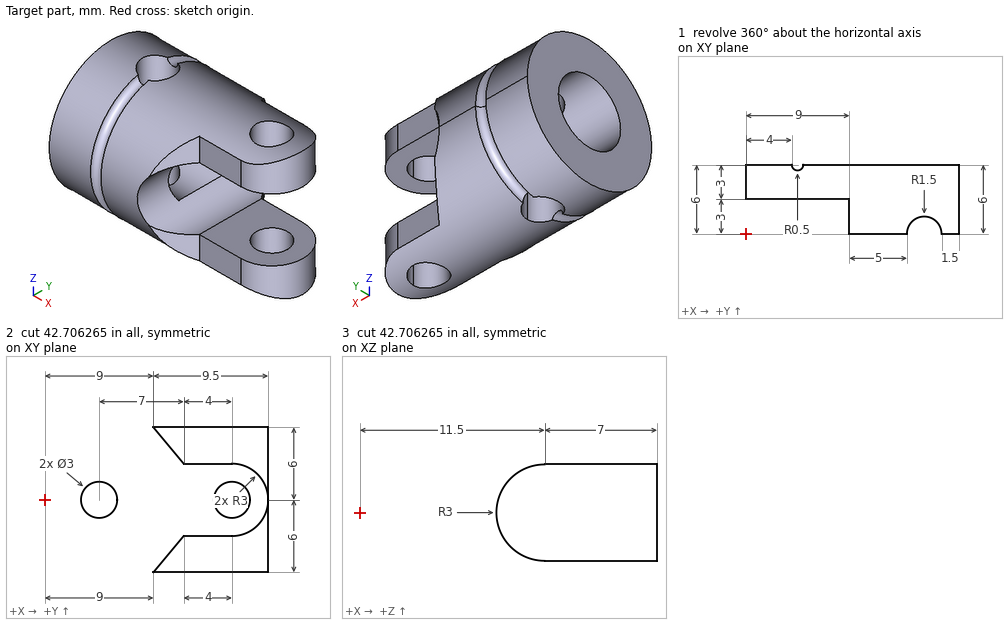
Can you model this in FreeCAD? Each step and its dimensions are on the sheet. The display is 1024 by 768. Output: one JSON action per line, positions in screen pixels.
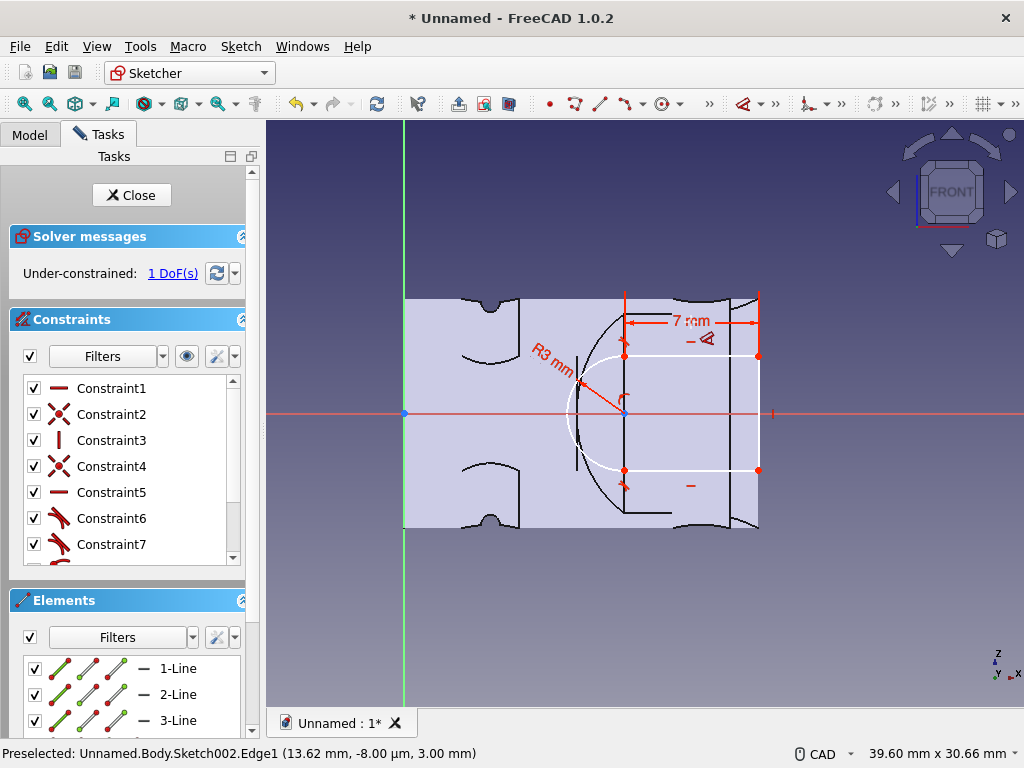
{"action": "left_click", "coordinate": [625, 356]}
{"action": "left_click", "coordinate": [515, 322]}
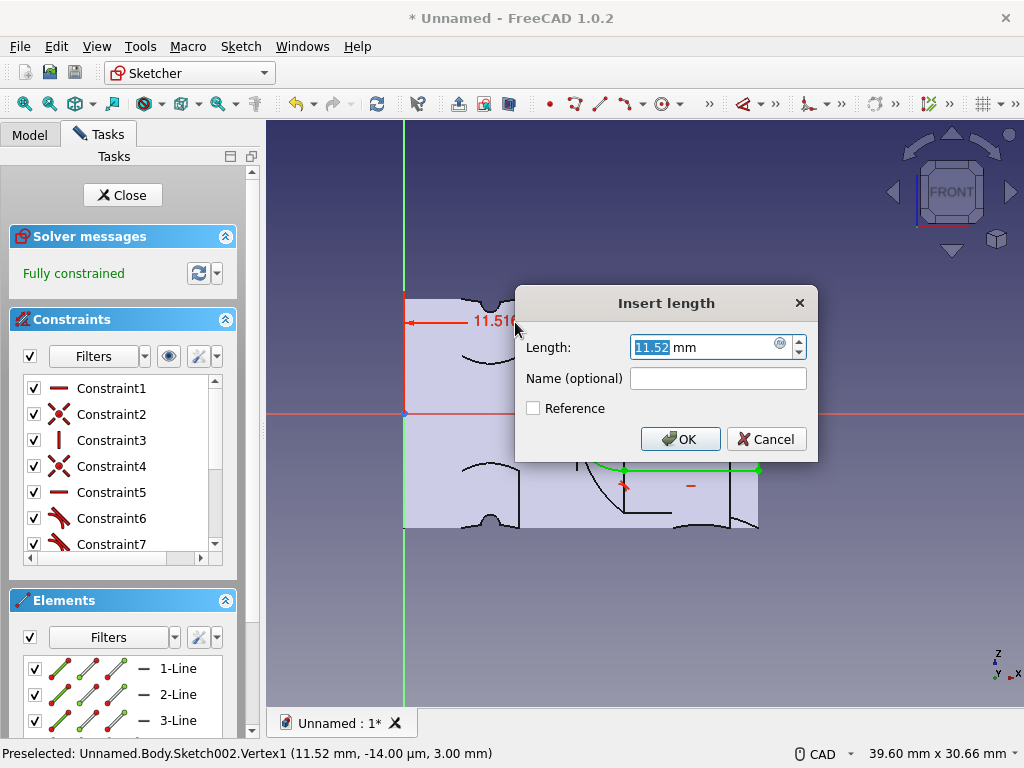
{"action": "type", "text": "11.5"}
{"action": "key", "text": "Return"}
{"action": "key", "text": "Escape"}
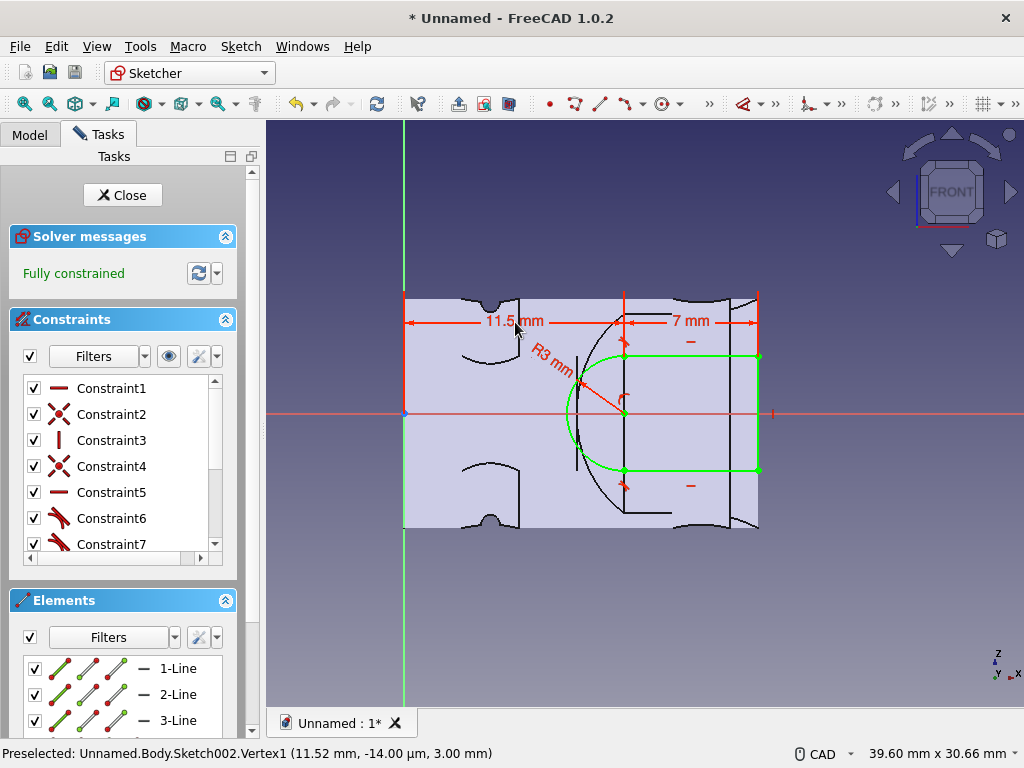
{"action": "left_click", "coordinate": [123, 195]}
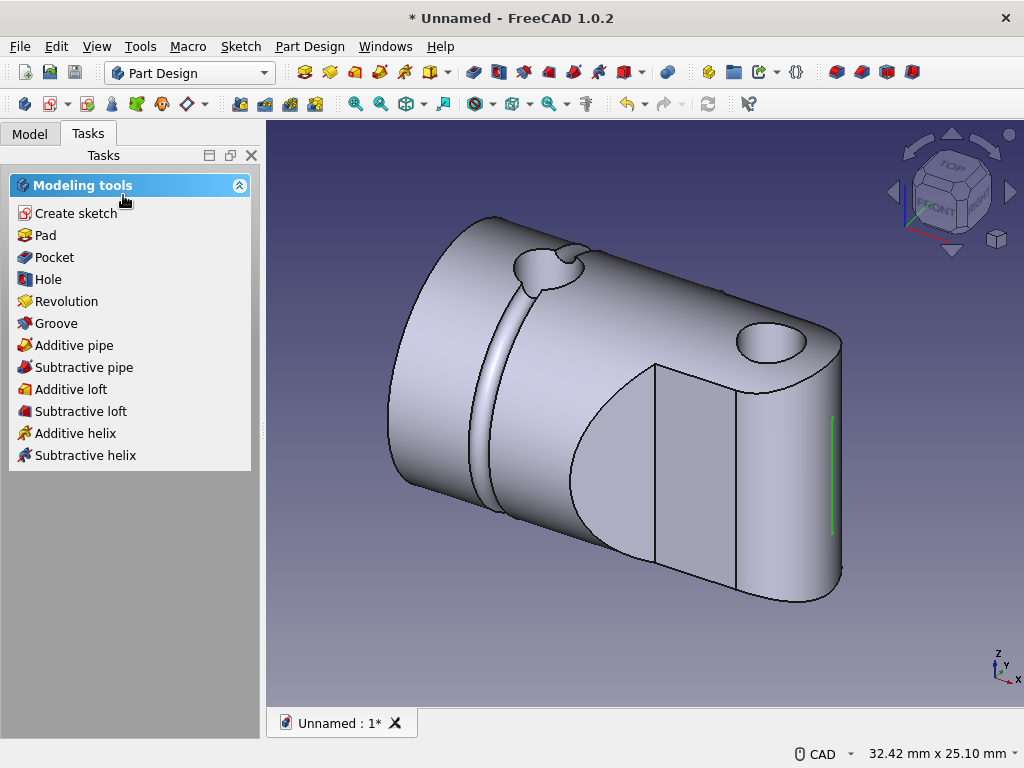
{"action": "left_click", "coordinate": [474, 72]}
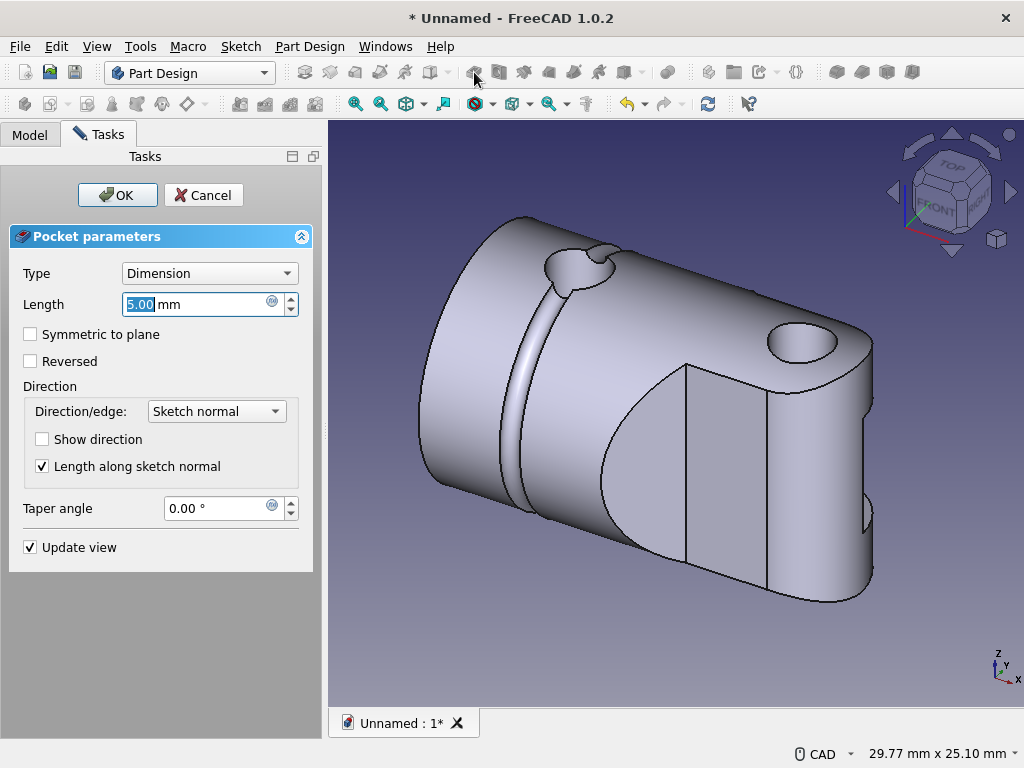
{"action": "type", "text": "42.706265"}
{"action": "key", "text": "Tab"}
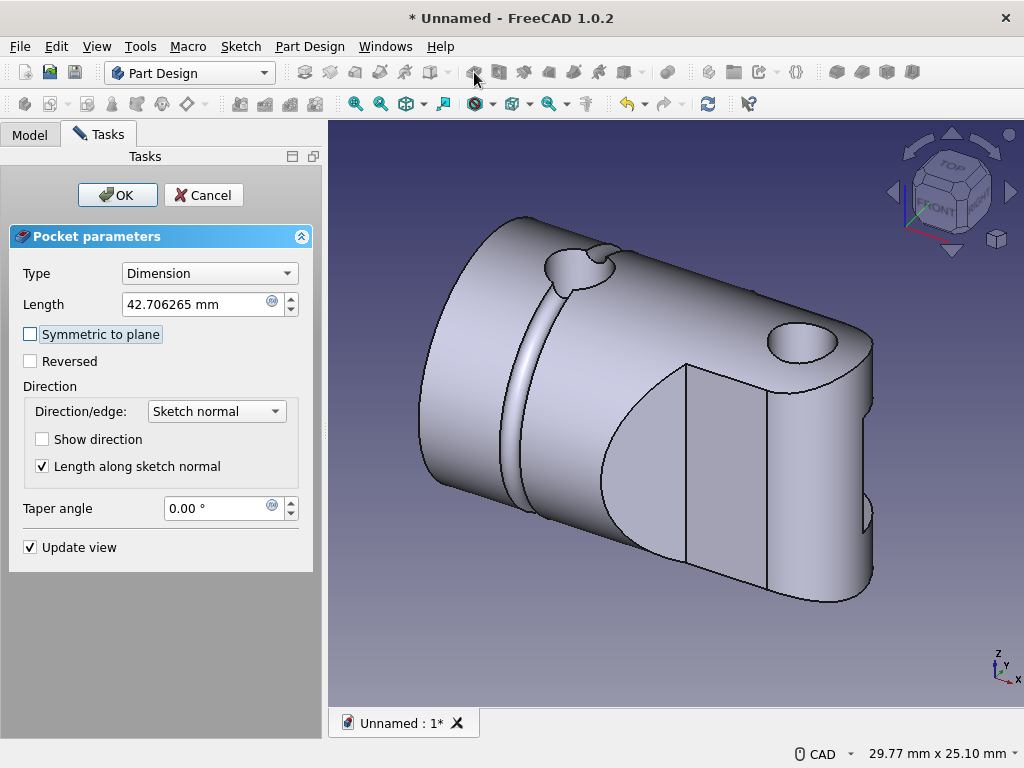
{"action": "left_click", "coordinate": [31, 334]}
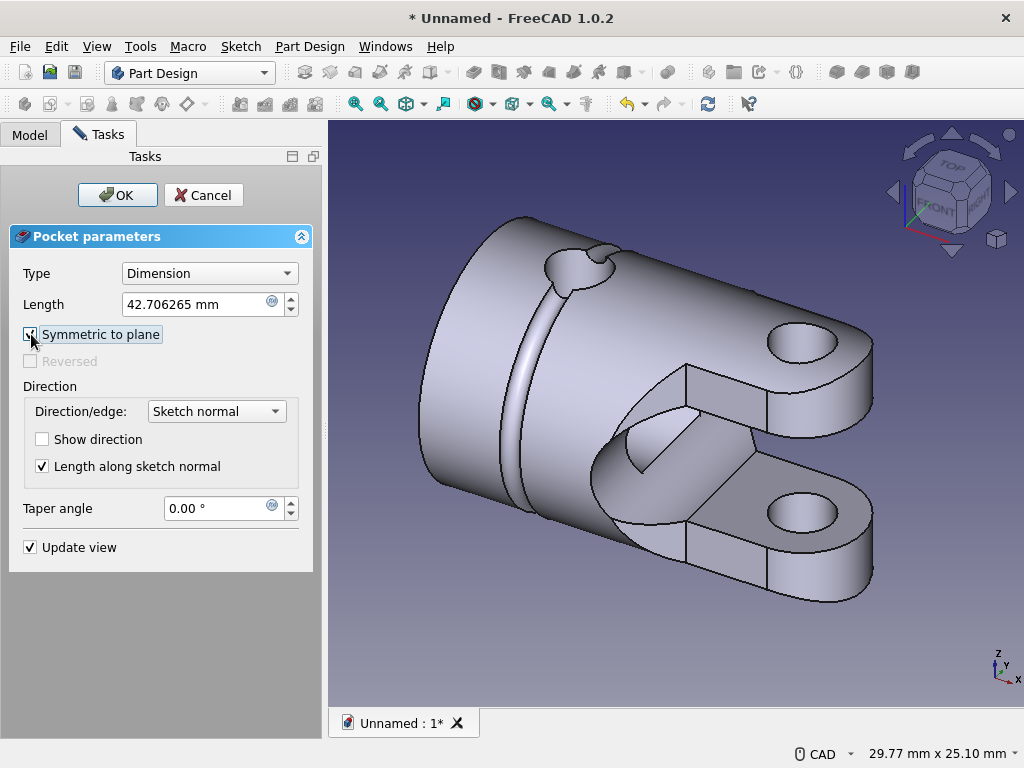
{"action": "left_click", "coordinate": [118, 195]}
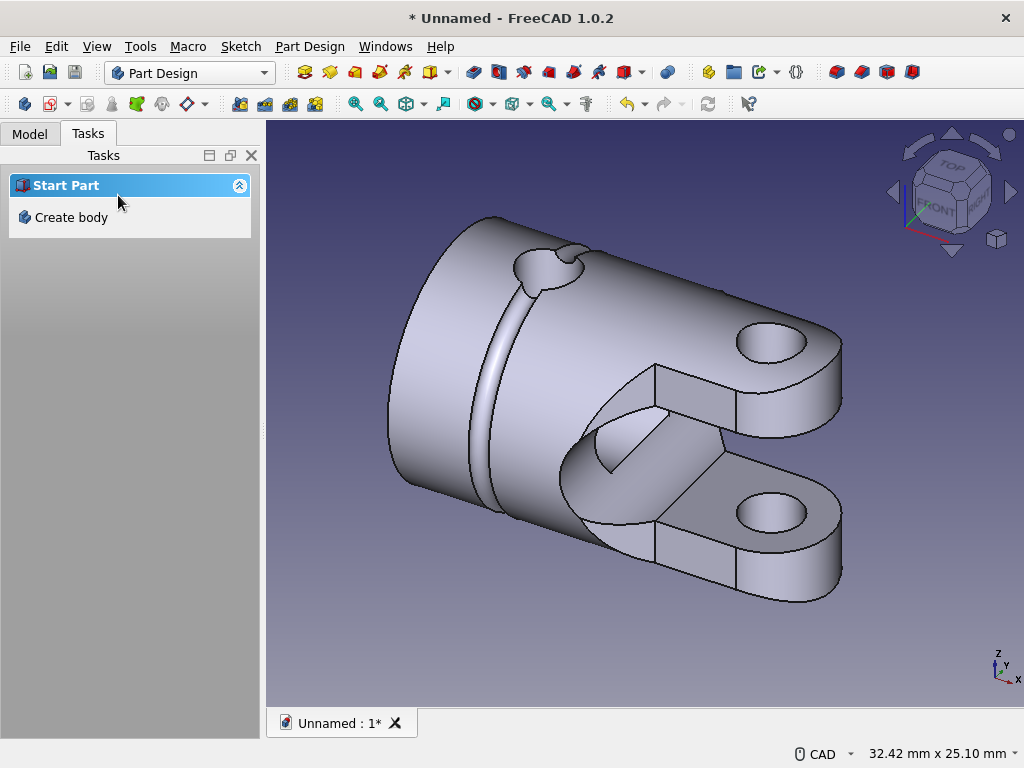
{"action": "key", "text": "0"}